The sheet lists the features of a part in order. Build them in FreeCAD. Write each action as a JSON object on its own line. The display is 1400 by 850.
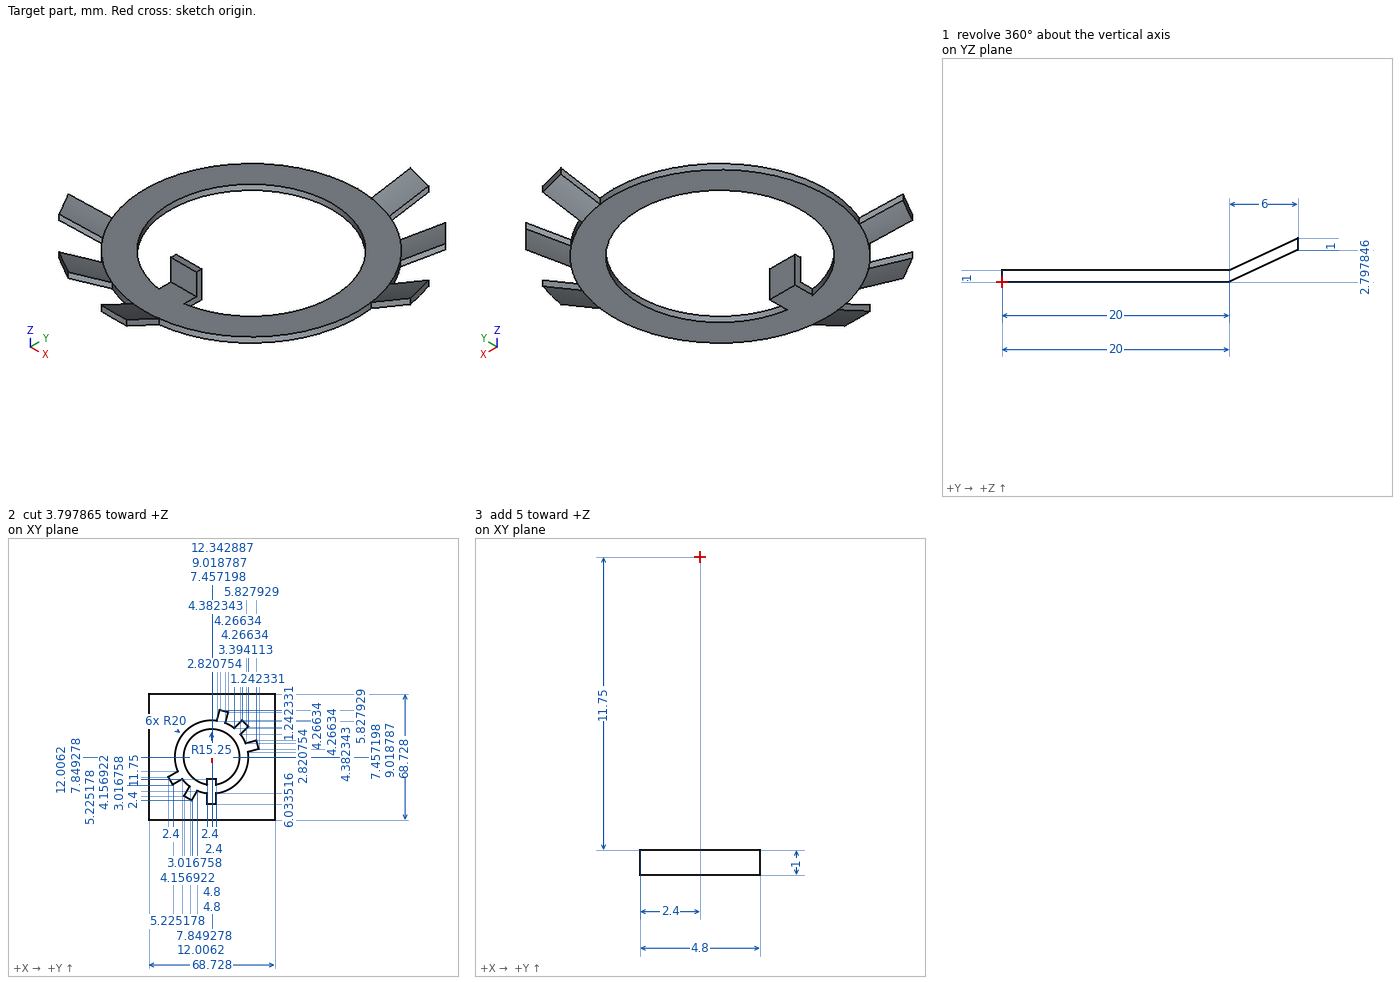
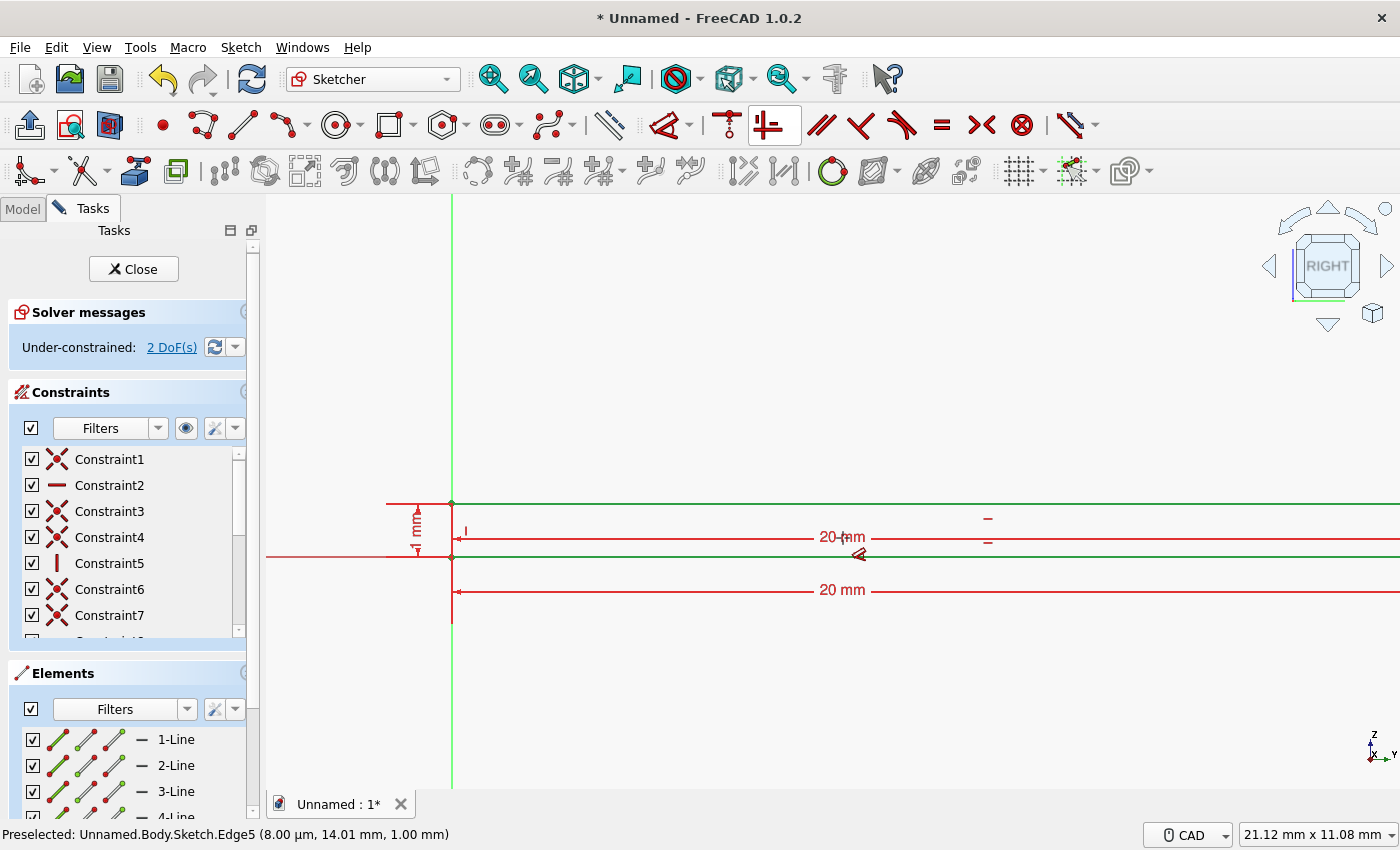
{"action": "scroll", "coordinate": [450, 521], "scroll_direction": "down", "scroll_amount": 4}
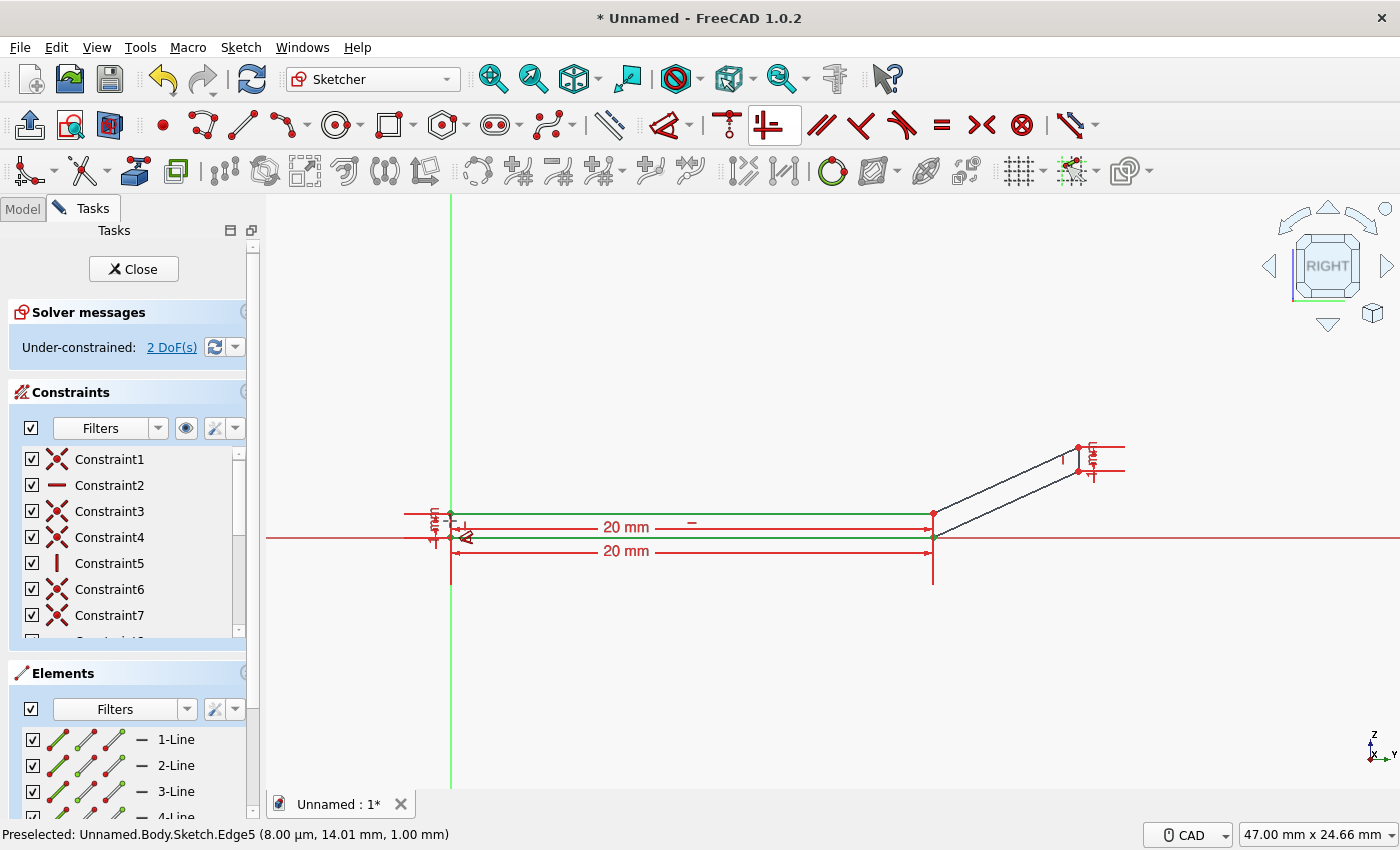
{"action": "left_click", "coordinate": [977, 518]}
{"action": "left_click", "coordinate": [1006, 572]}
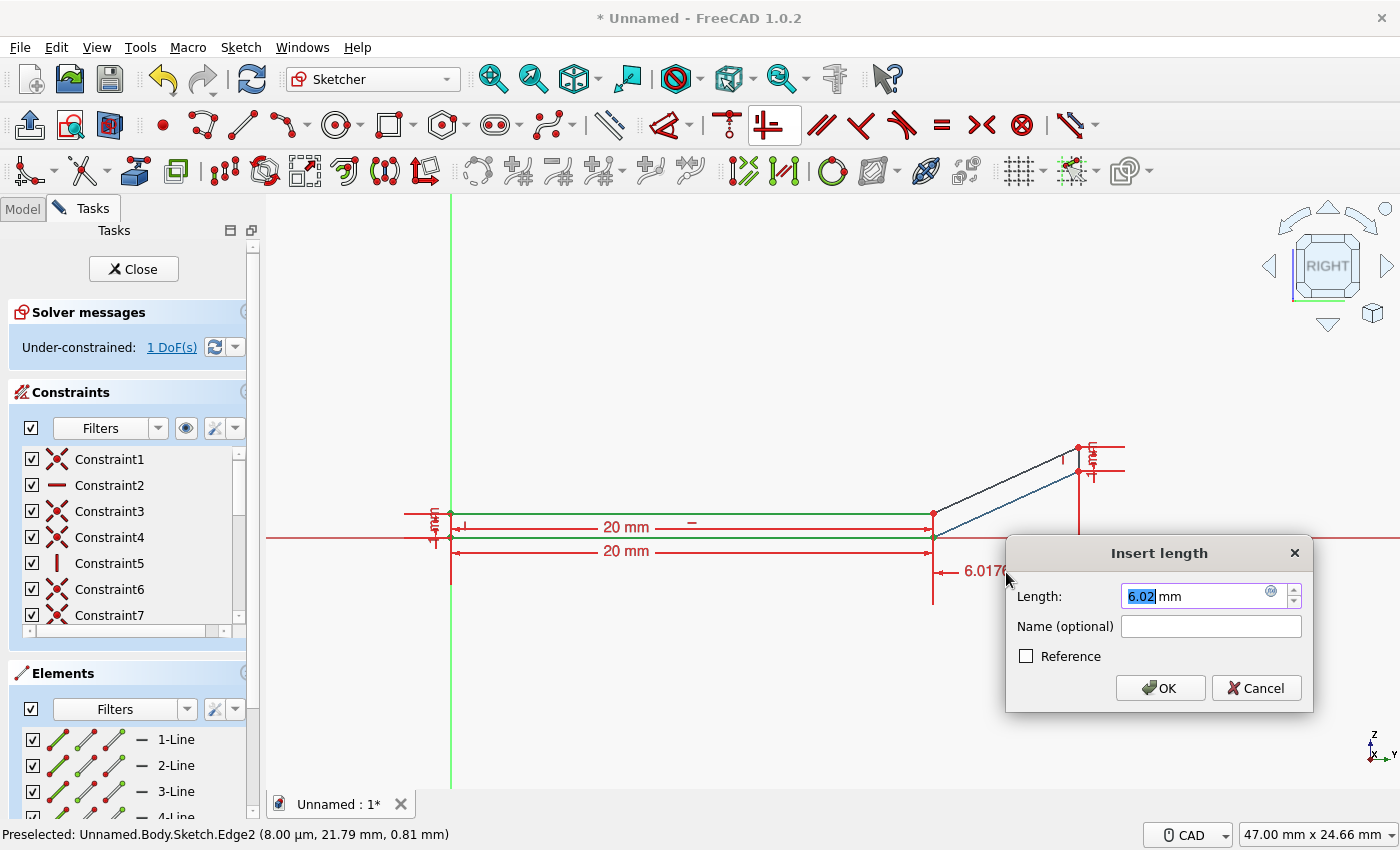
{"action": "type", "text": "6"}
{"action": "key", "text": "Return"}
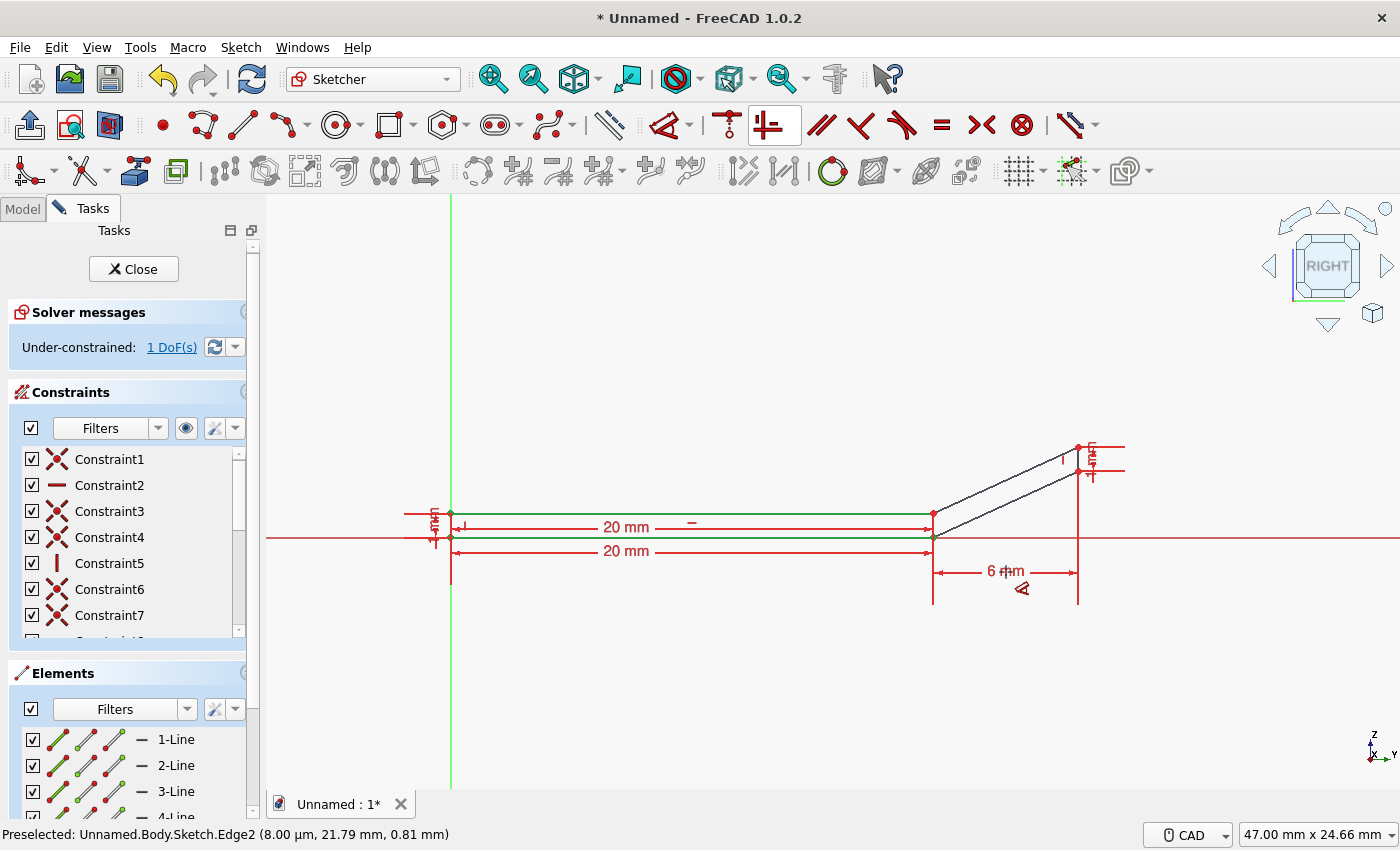
{"action": "left_click", "coordinate": [1078, 471]}
{"action": "left_click", "coordinate": [1112, 505]}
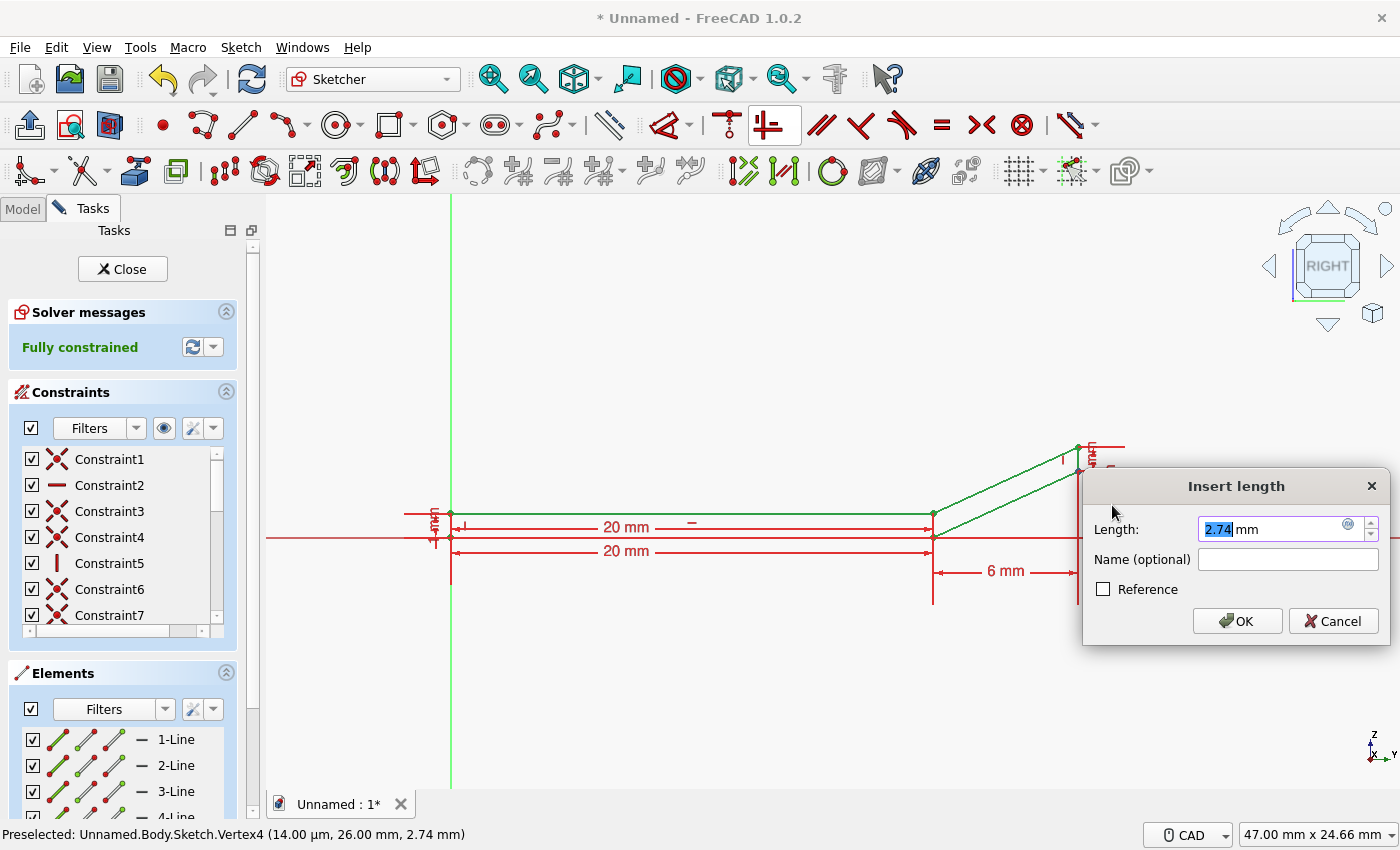
{"action": "type", "text": "2.797846"}
{"action": "key", "text": "Return"}
{"action": "key", "text": "Escape"}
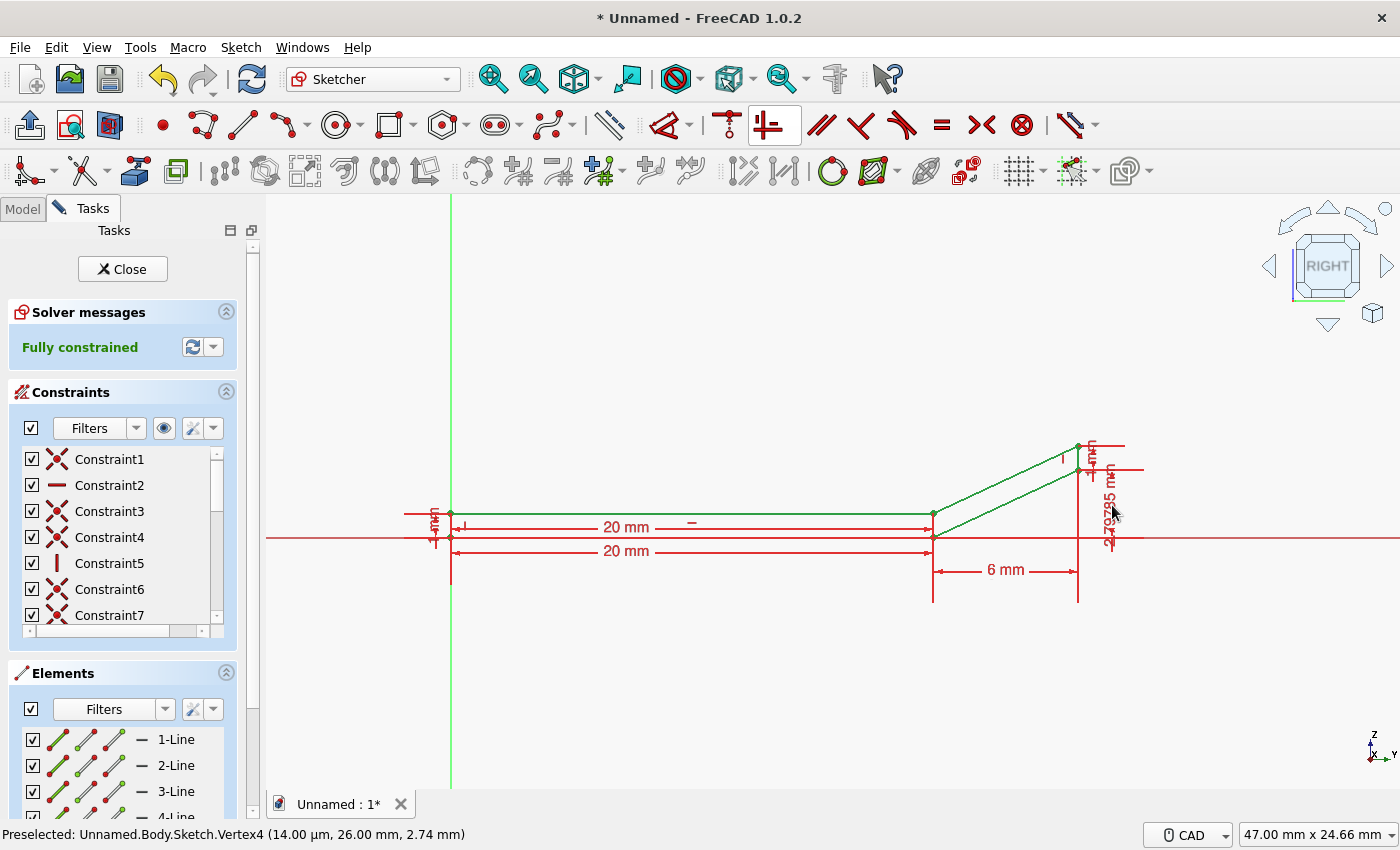
{"action": "left_click", "coordinate": [123, 269]}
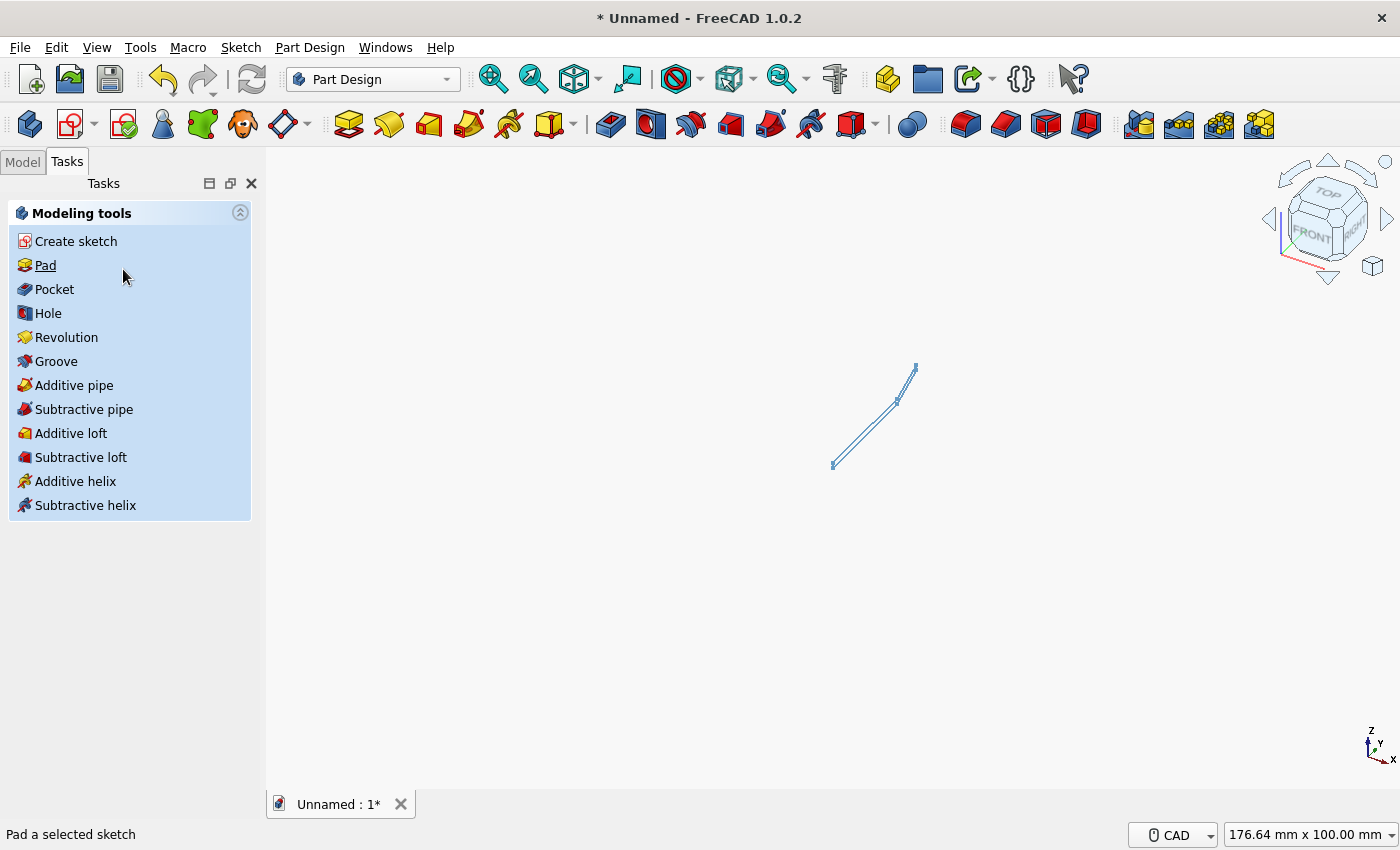
{"action": "left_click", "coordinate": [390, 124]}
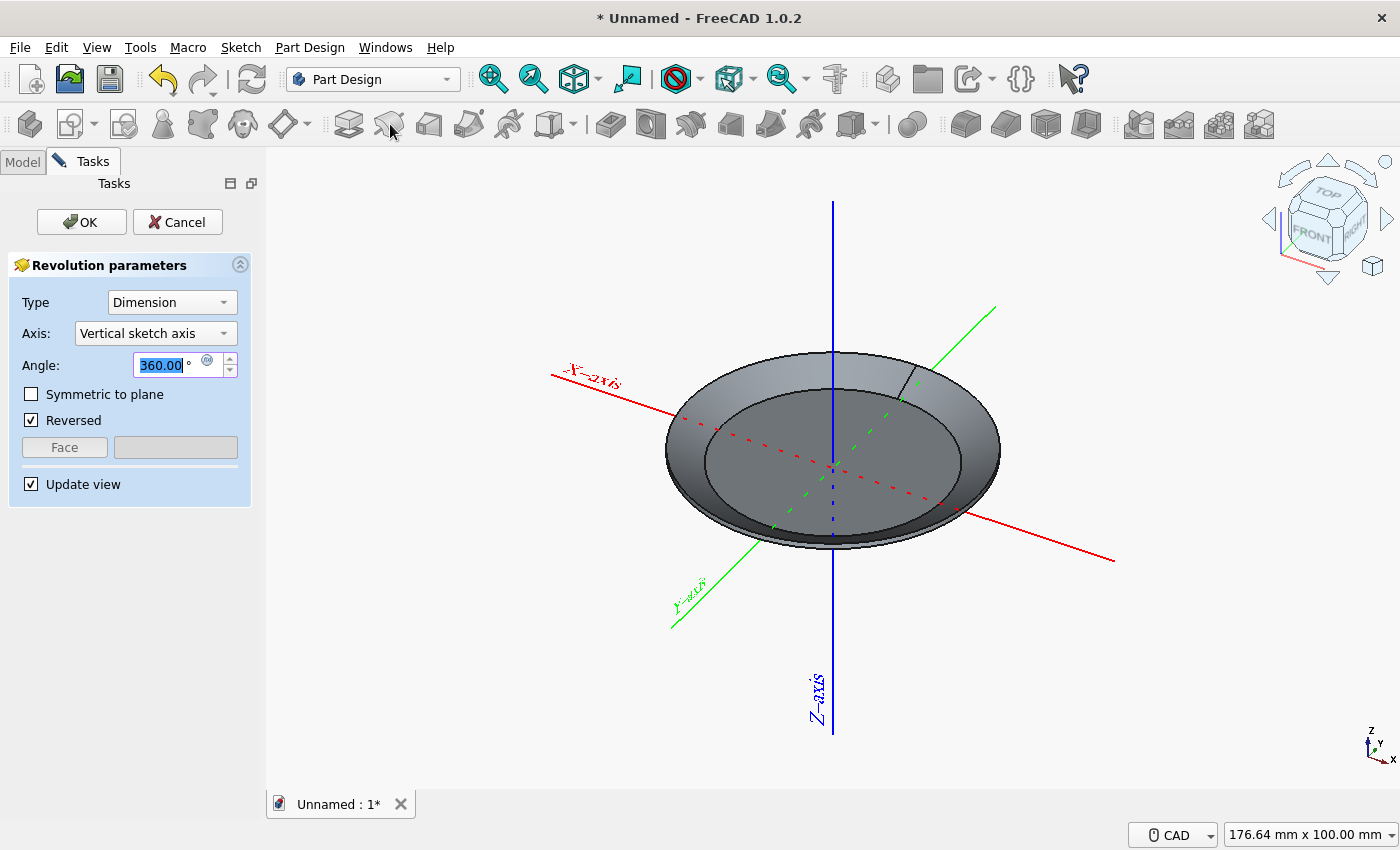
{"action": "left_click", "coordinate": [82, 222]}